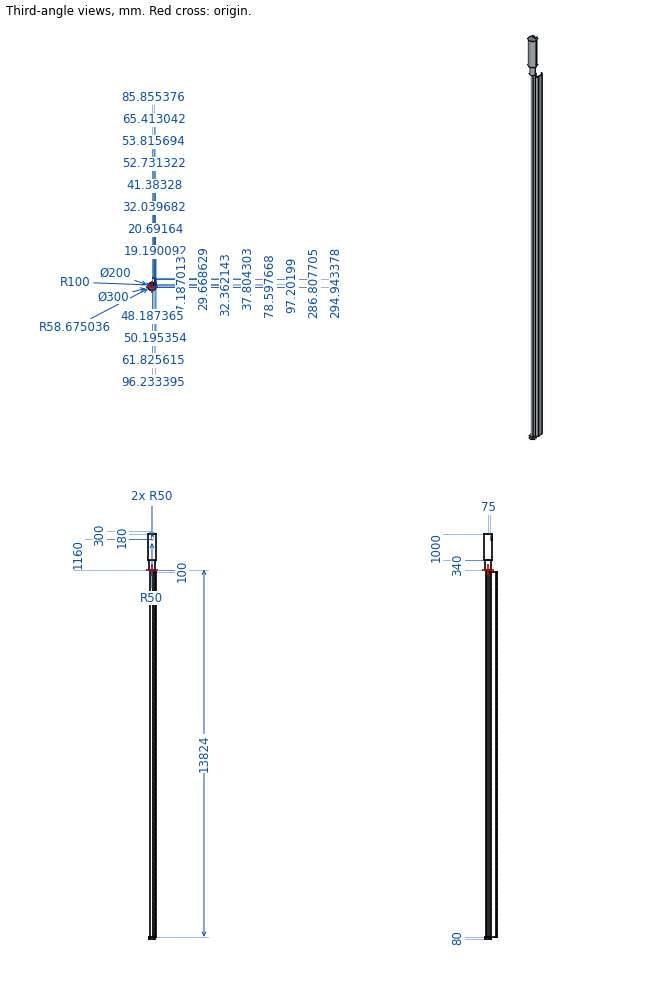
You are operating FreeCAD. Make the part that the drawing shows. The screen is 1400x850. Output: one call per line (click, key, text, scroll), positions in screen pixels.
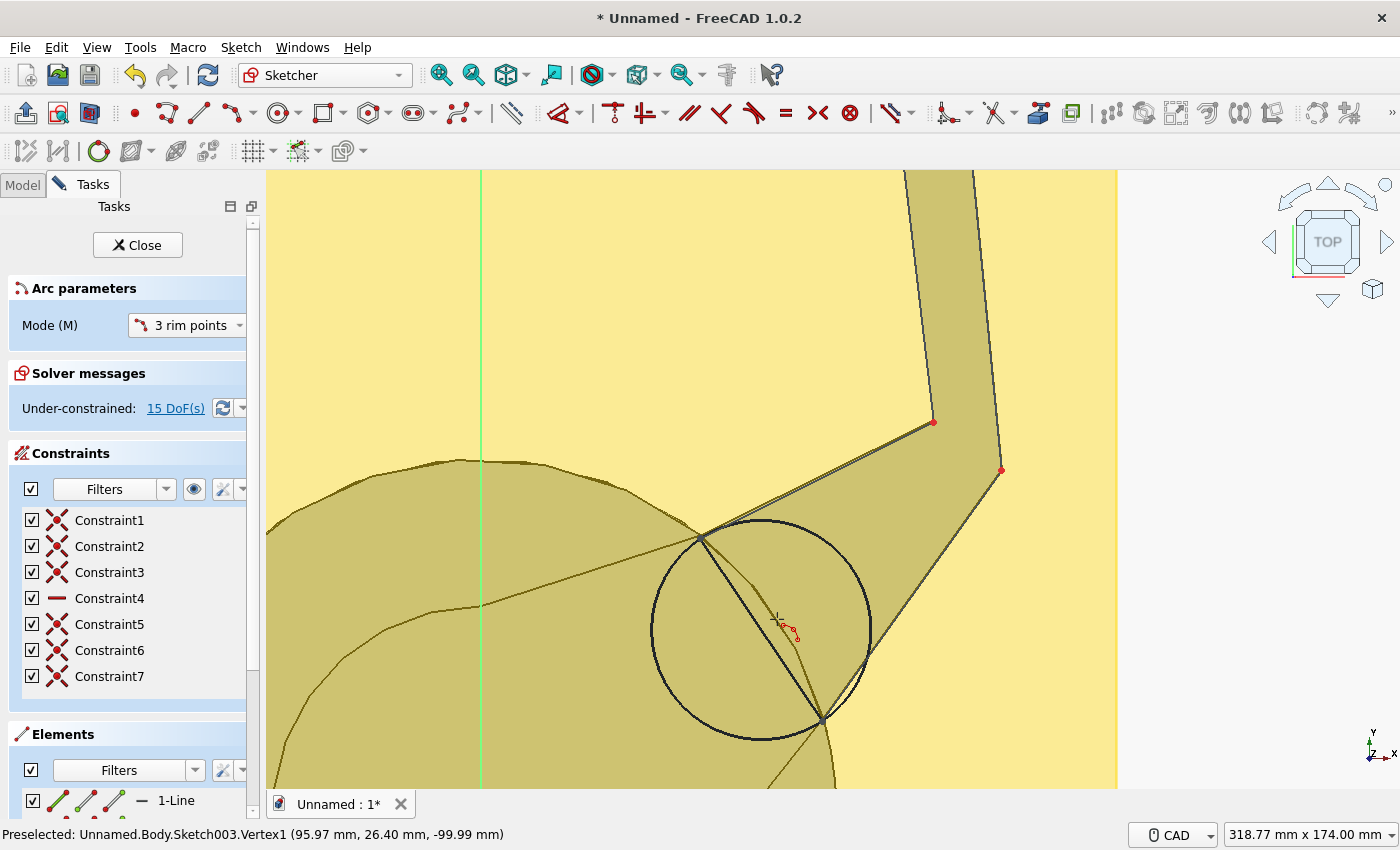
click(777, 617)
key(Escape)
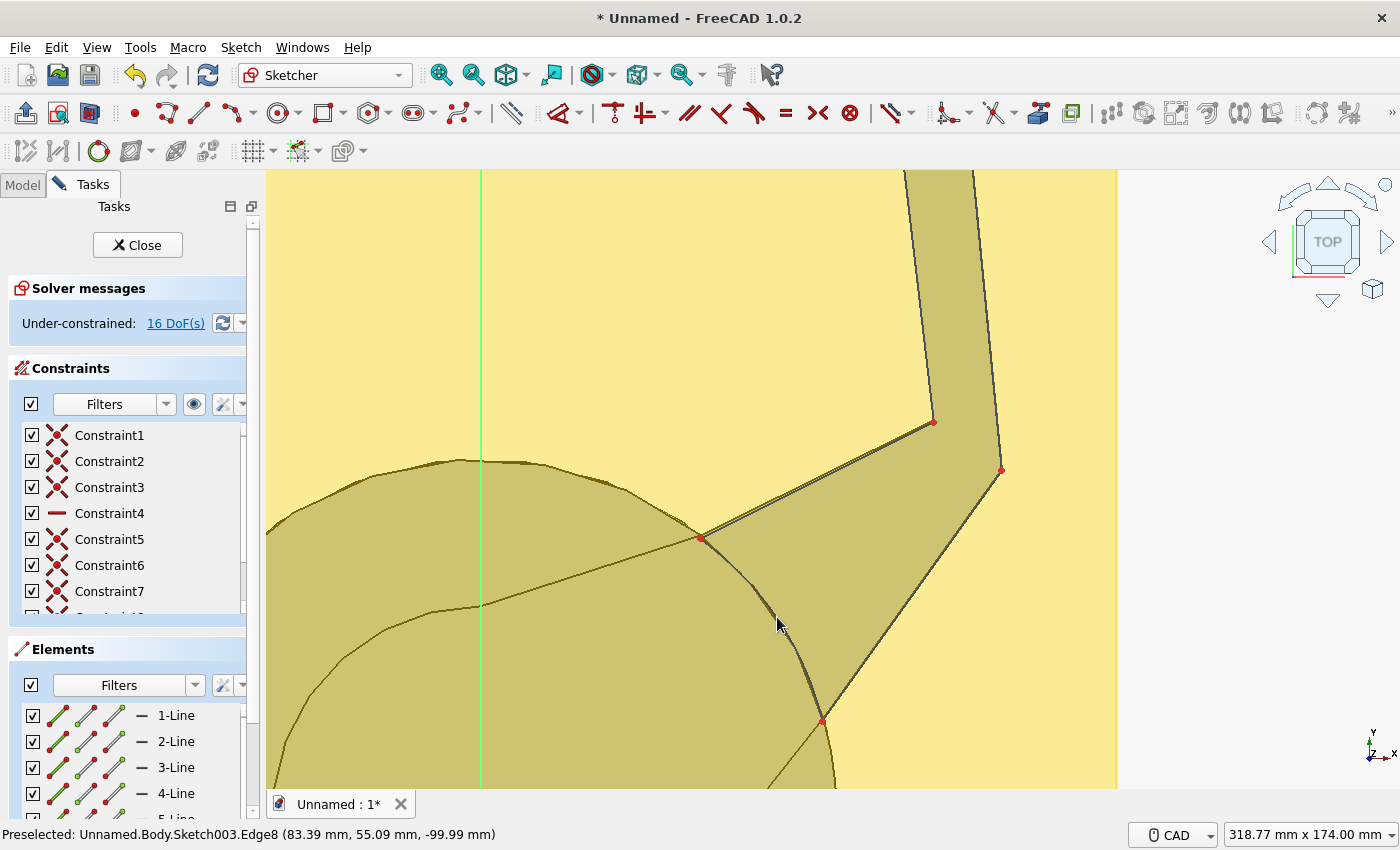
scroll(778, 620, down, 5)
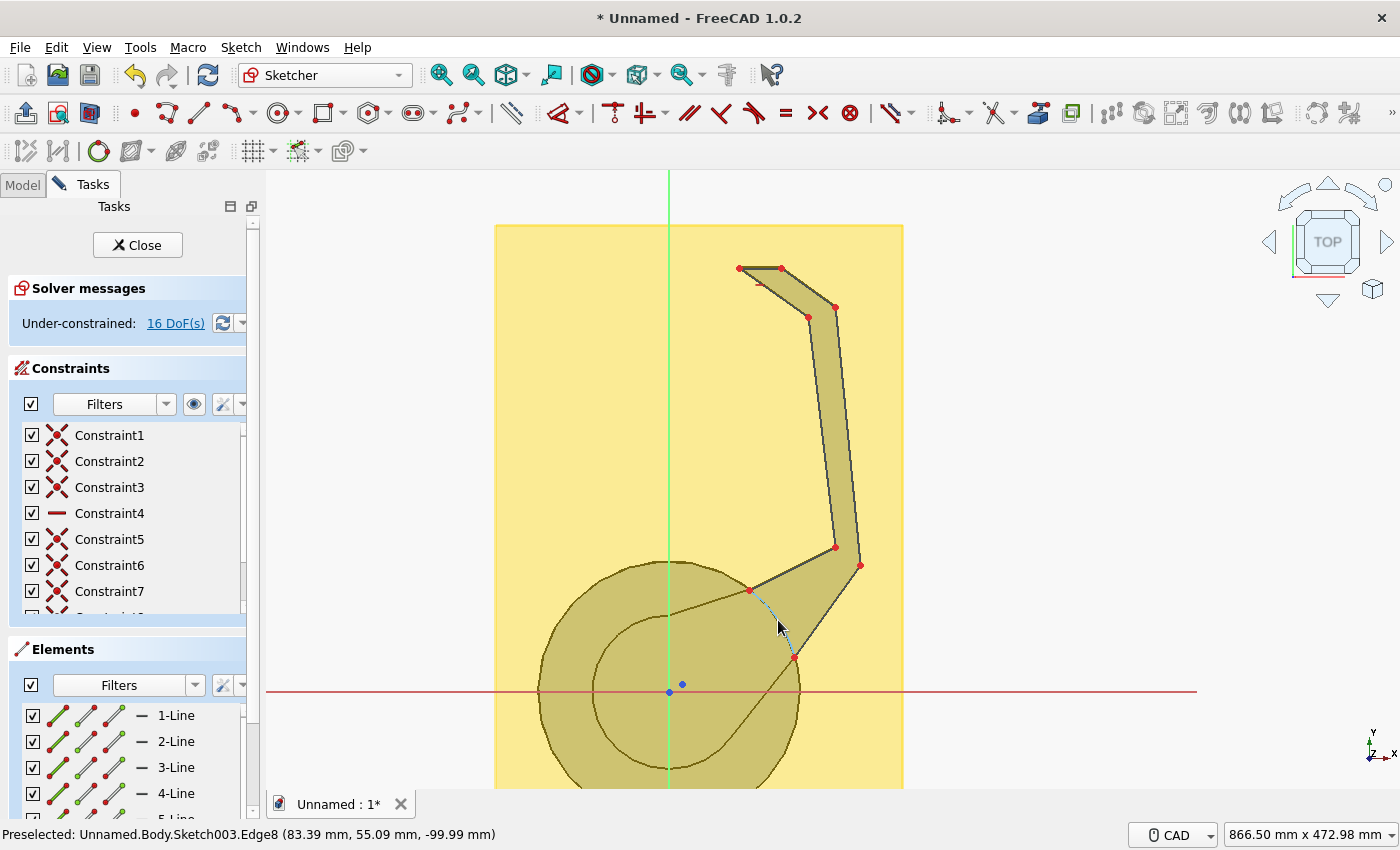
drag(659, 675, 692, 702)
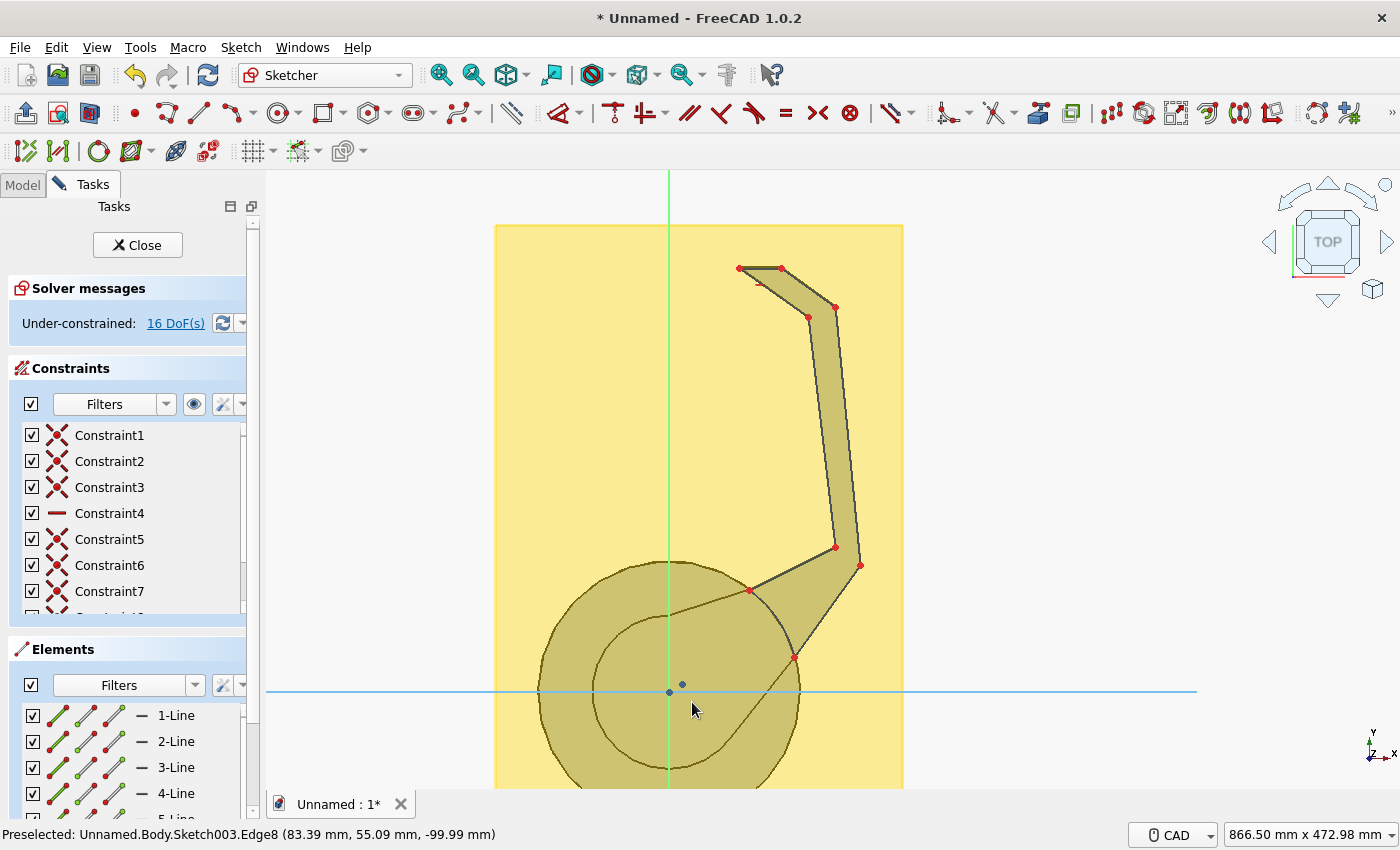
key(c)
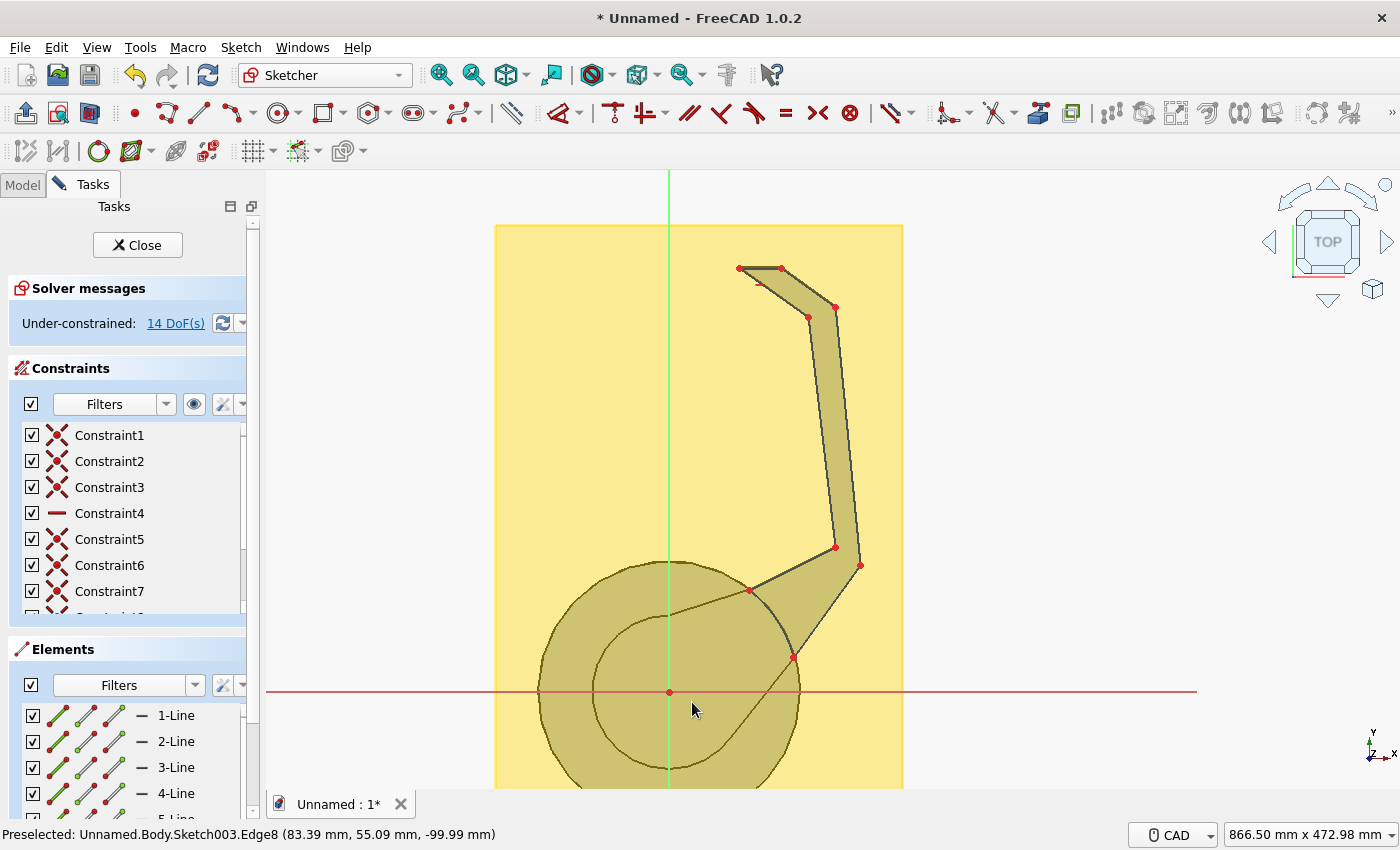
key(d)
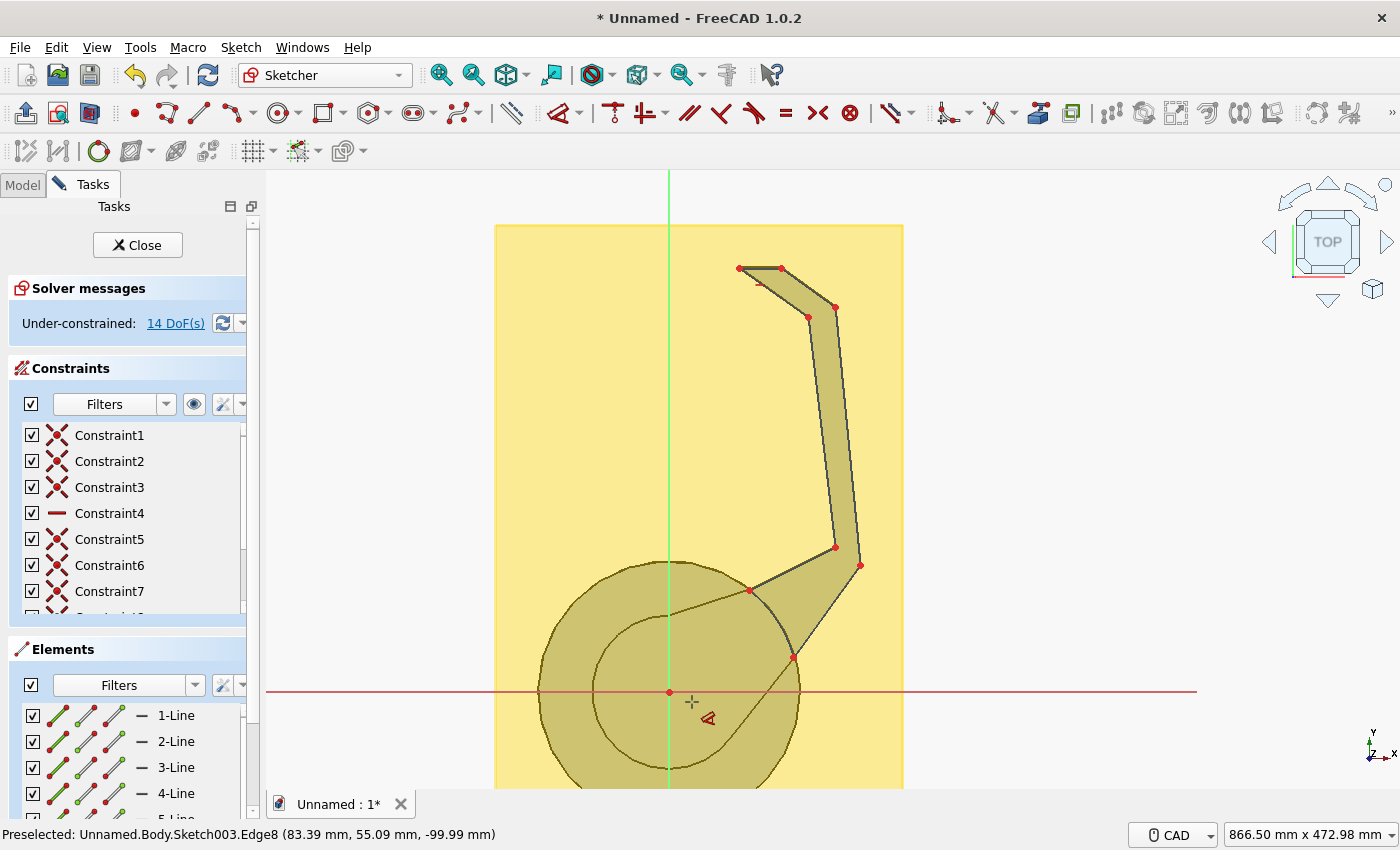
click(785, 635)
click(762, 560)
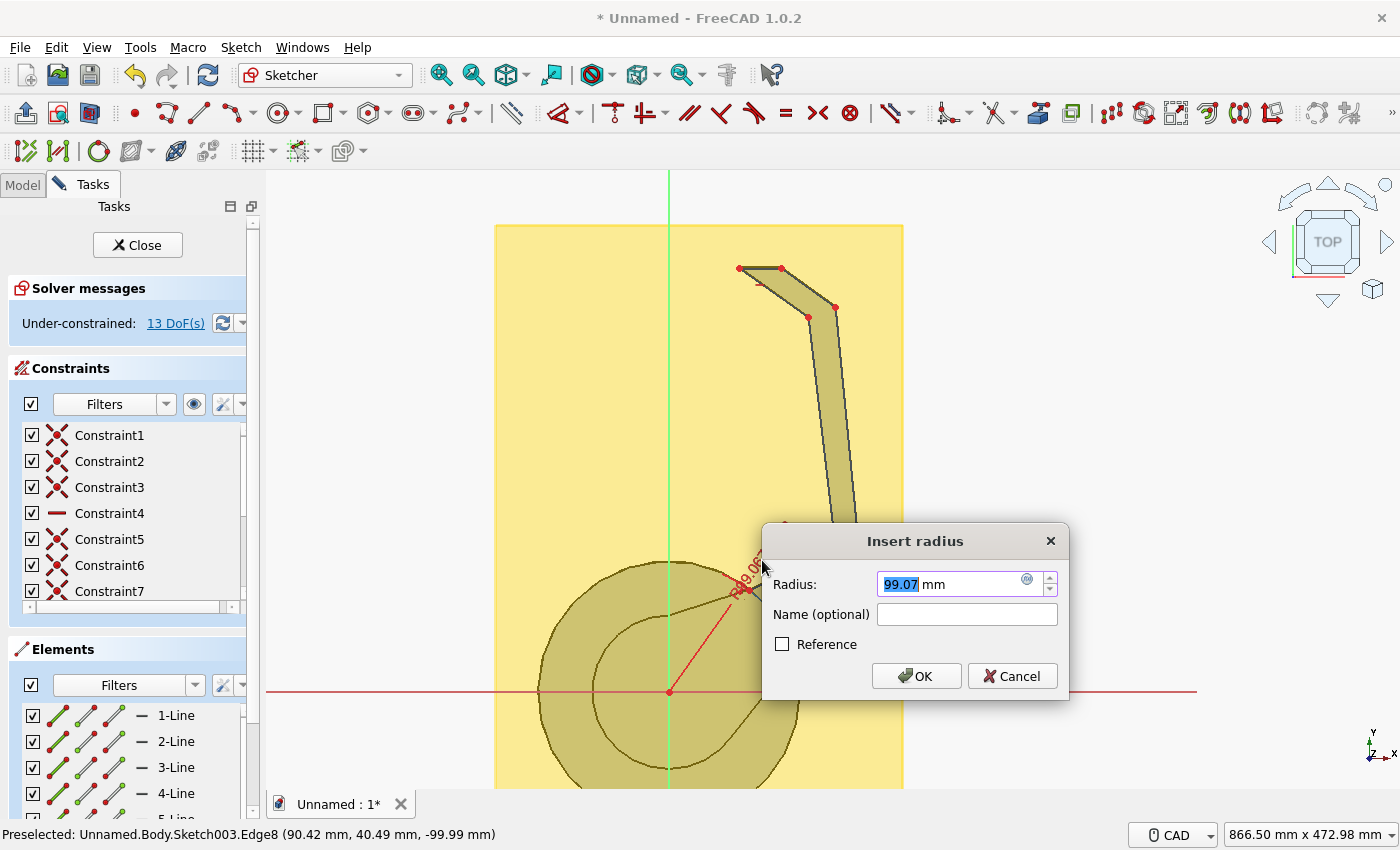
text(100)
key(Return)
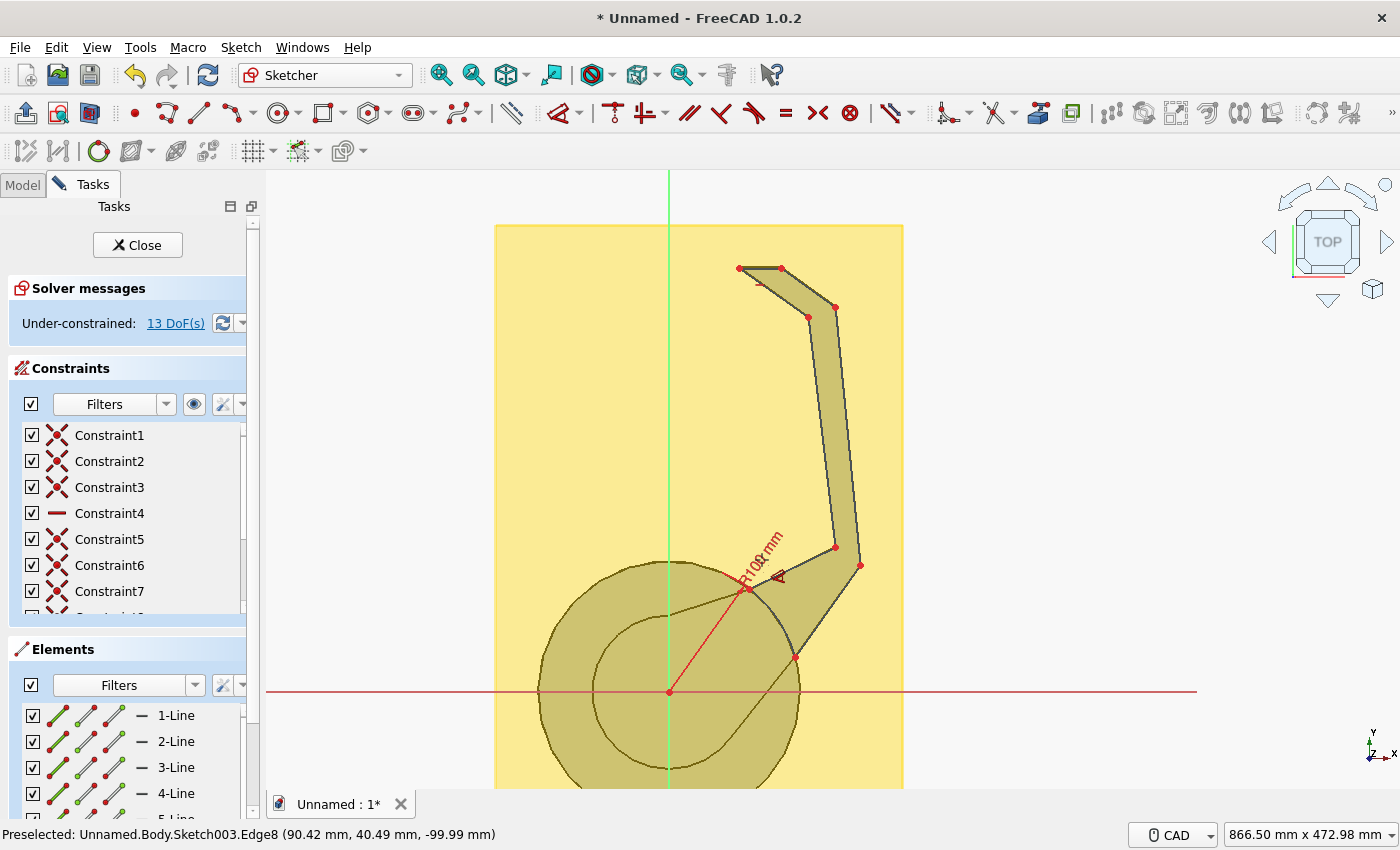
click(769, 269)
click(761, 235)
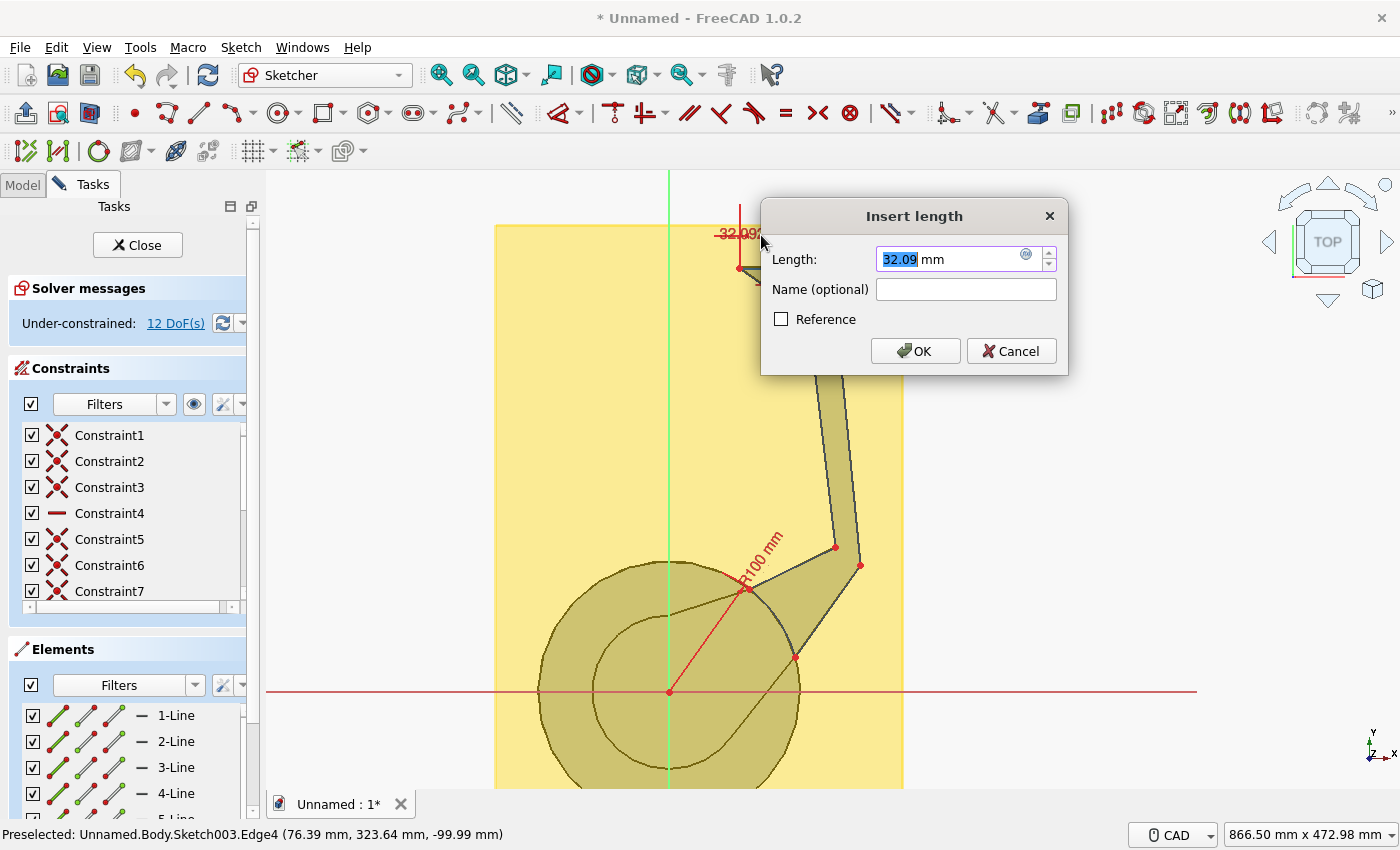
text(32.039682)
key(Return)